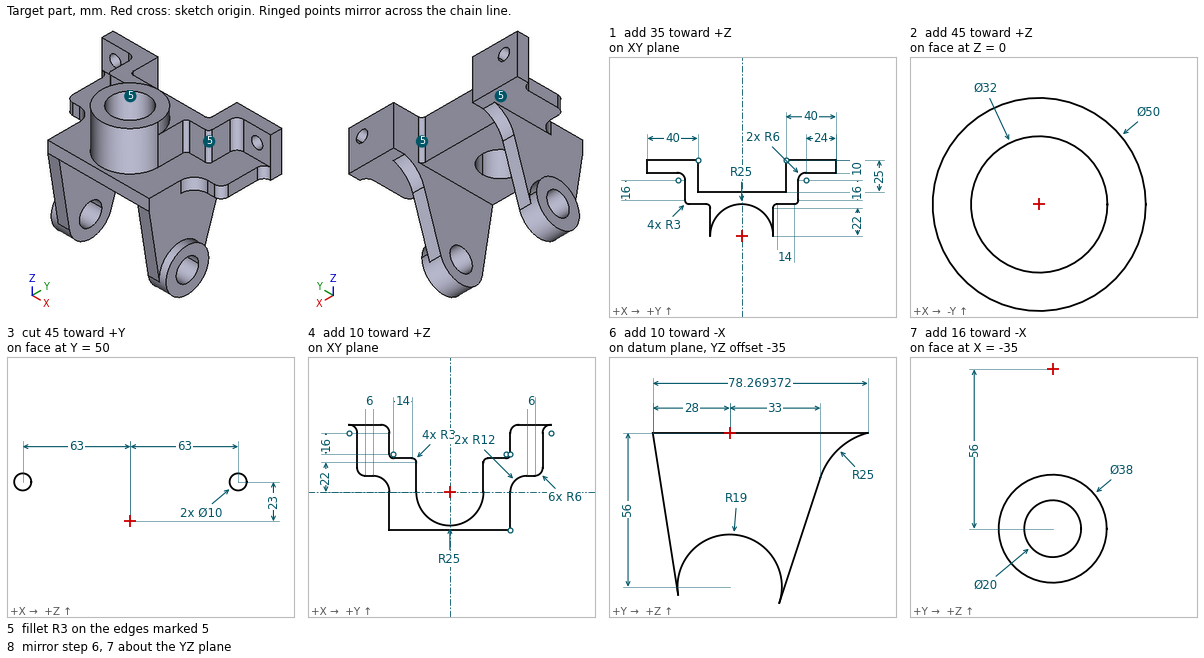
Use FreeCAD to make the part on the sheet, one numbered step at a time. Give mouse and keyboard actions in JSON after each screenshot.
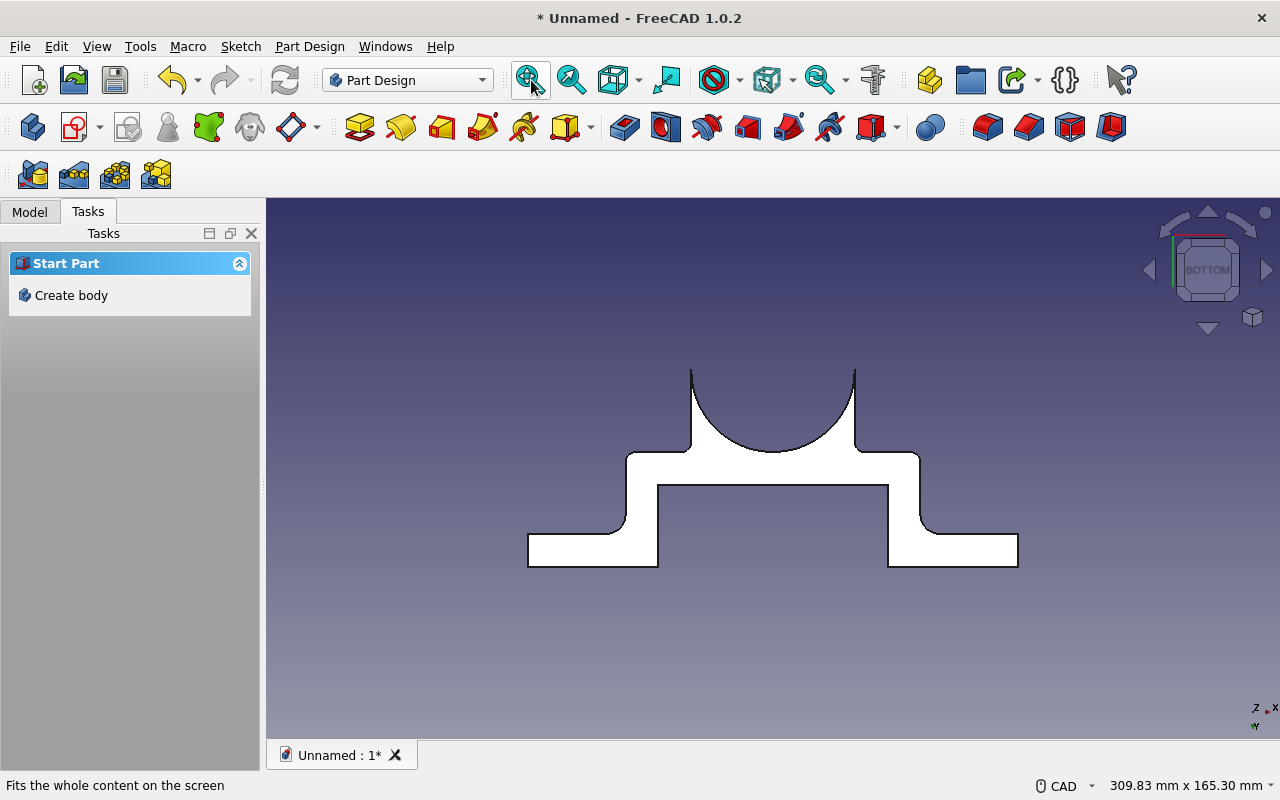
{"action": "left_click", "coordinate": [843, 467]}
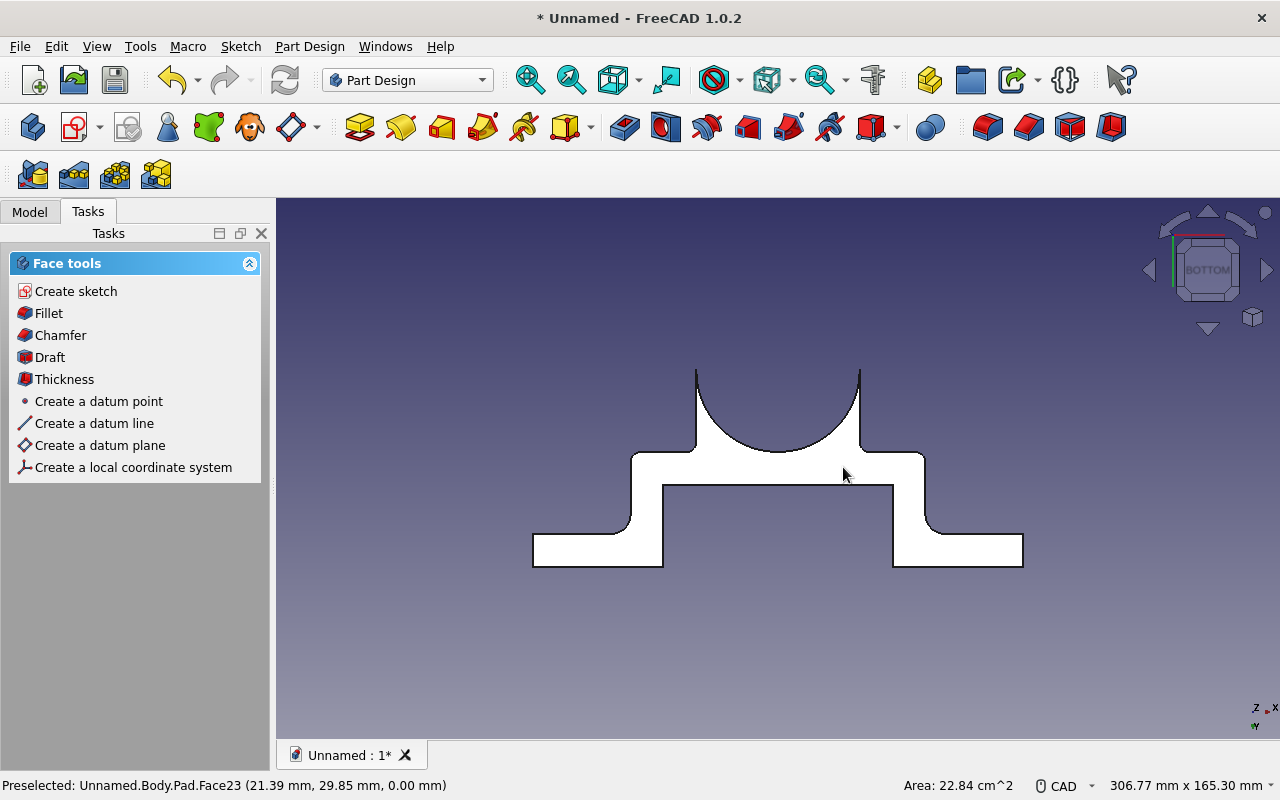
{"action": "left_click", "coordinate": [74, 128]}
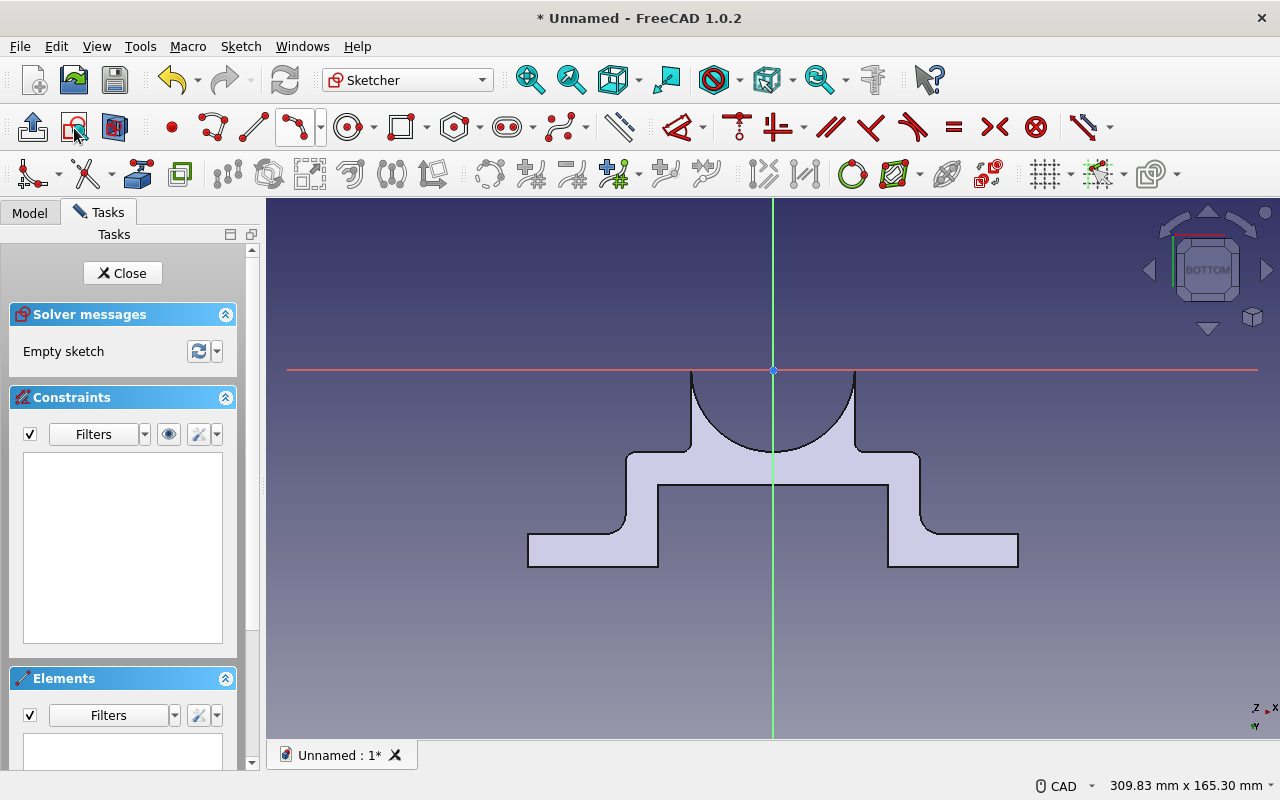
{"action": "scroll", "coordinate": [829, 290], "scroll_direction": "up", "scroll_amount": 4}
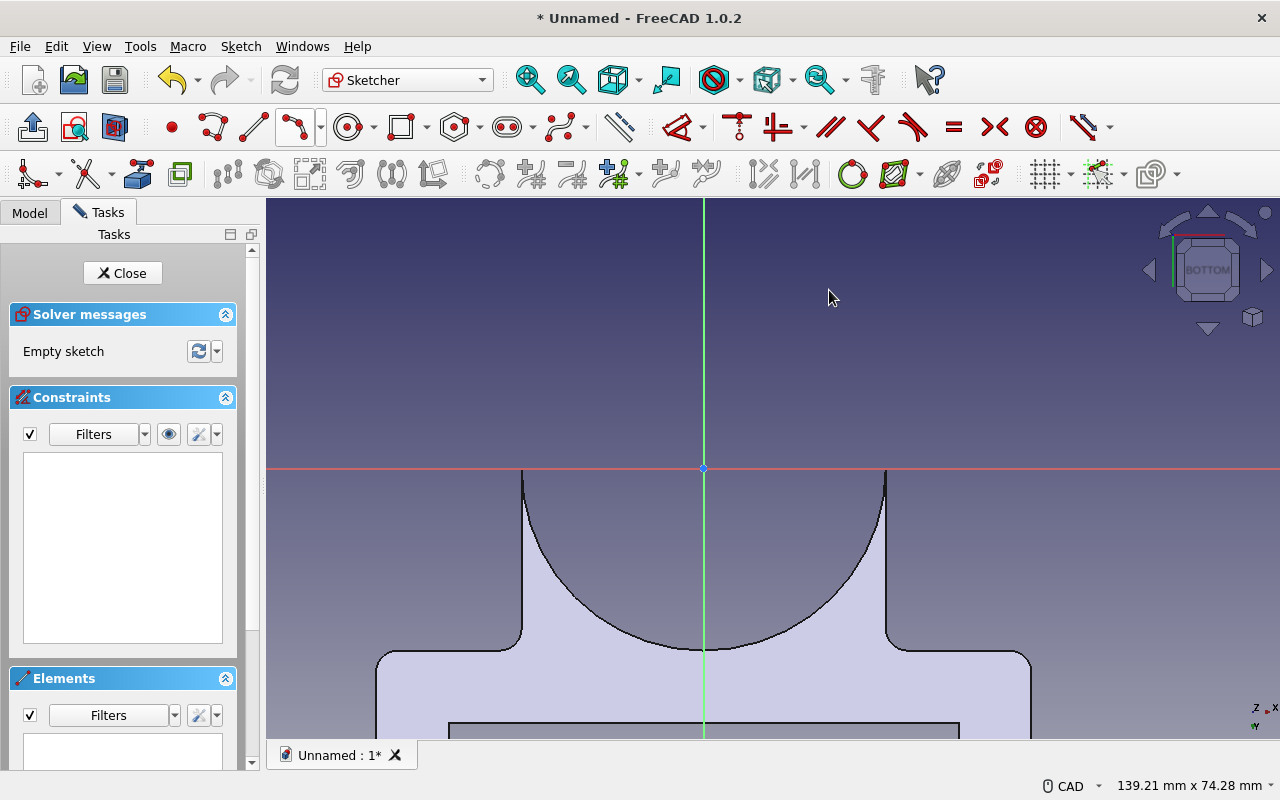
{"action": "left_click", "coordinate": [348, 128]}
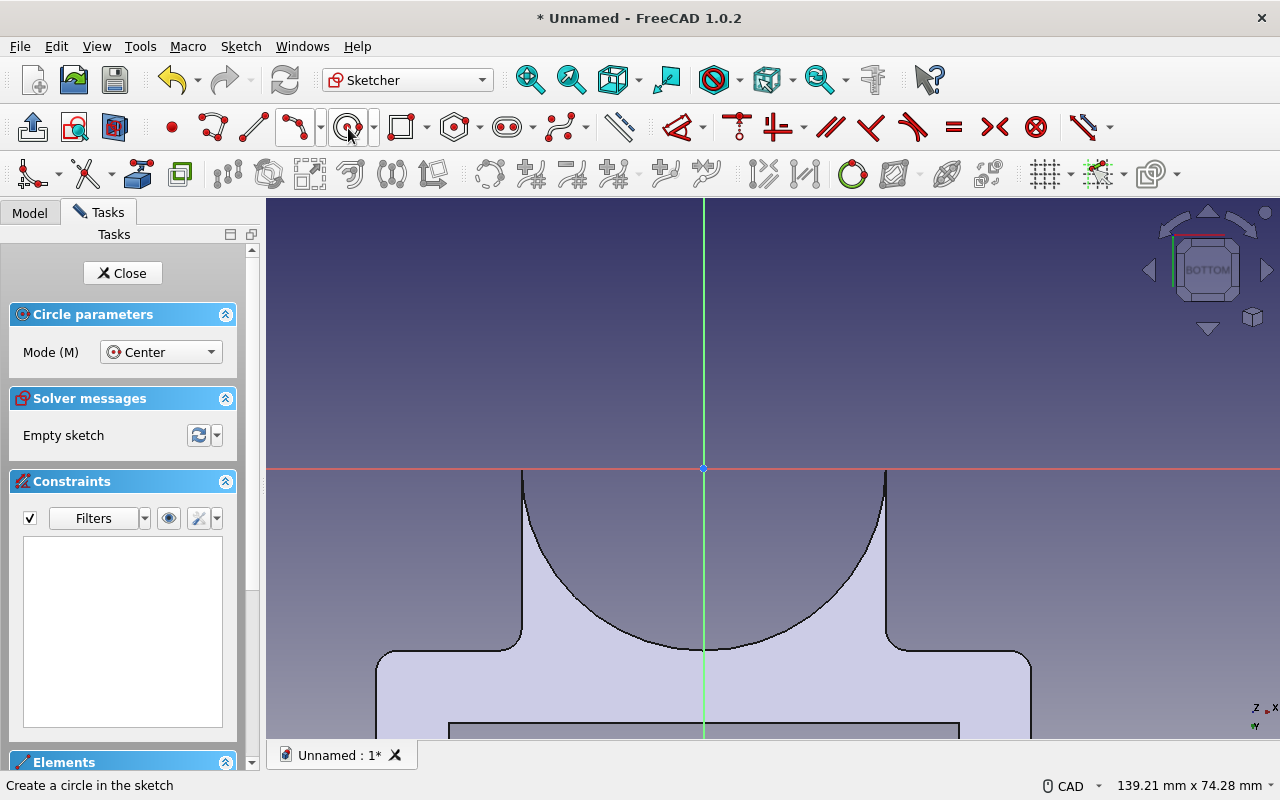
{"action": "left_click", "coordinate": [704, 469]}
{"action": "left_click", "coordinate": [832, 340]}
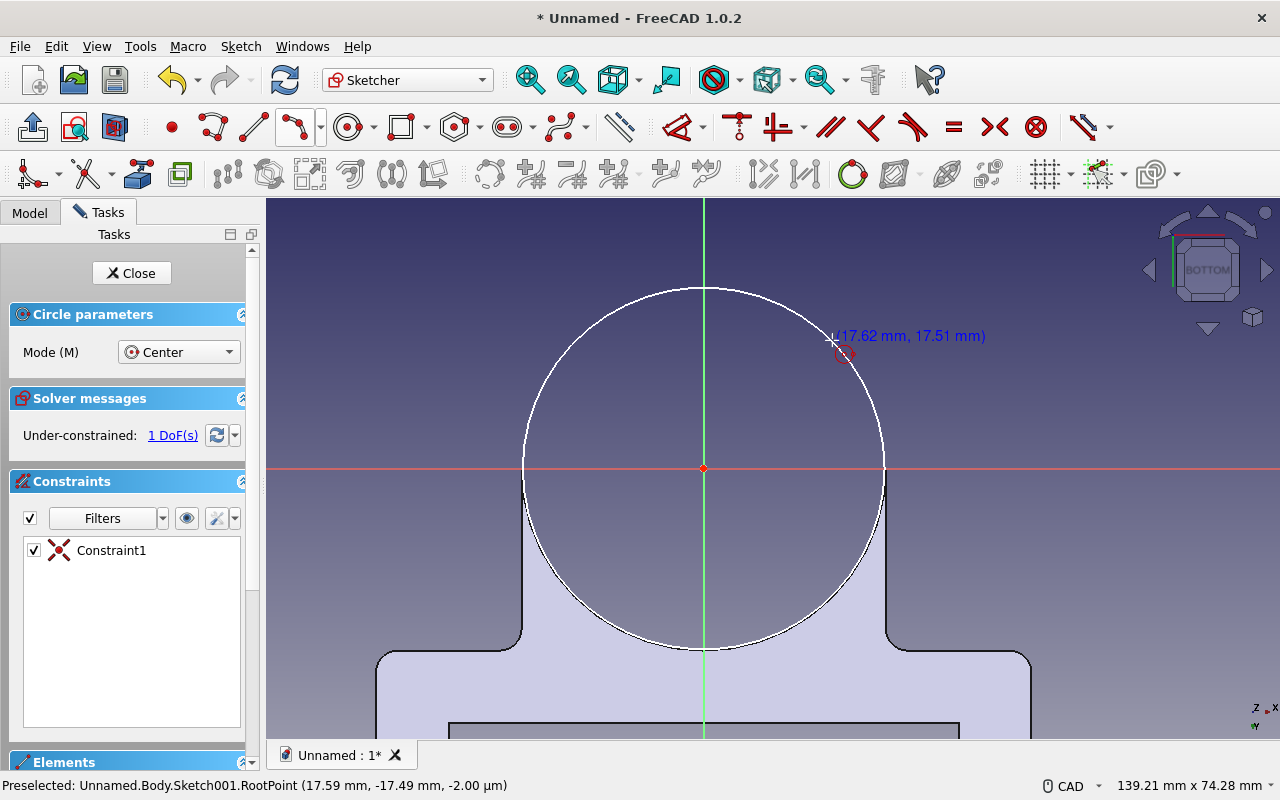
{"action": "left_click", "coordinate": [704, 469]}
{"action": "left_click", "coordinate": [786, 386]}
{"action": "key", "text": "Escape"}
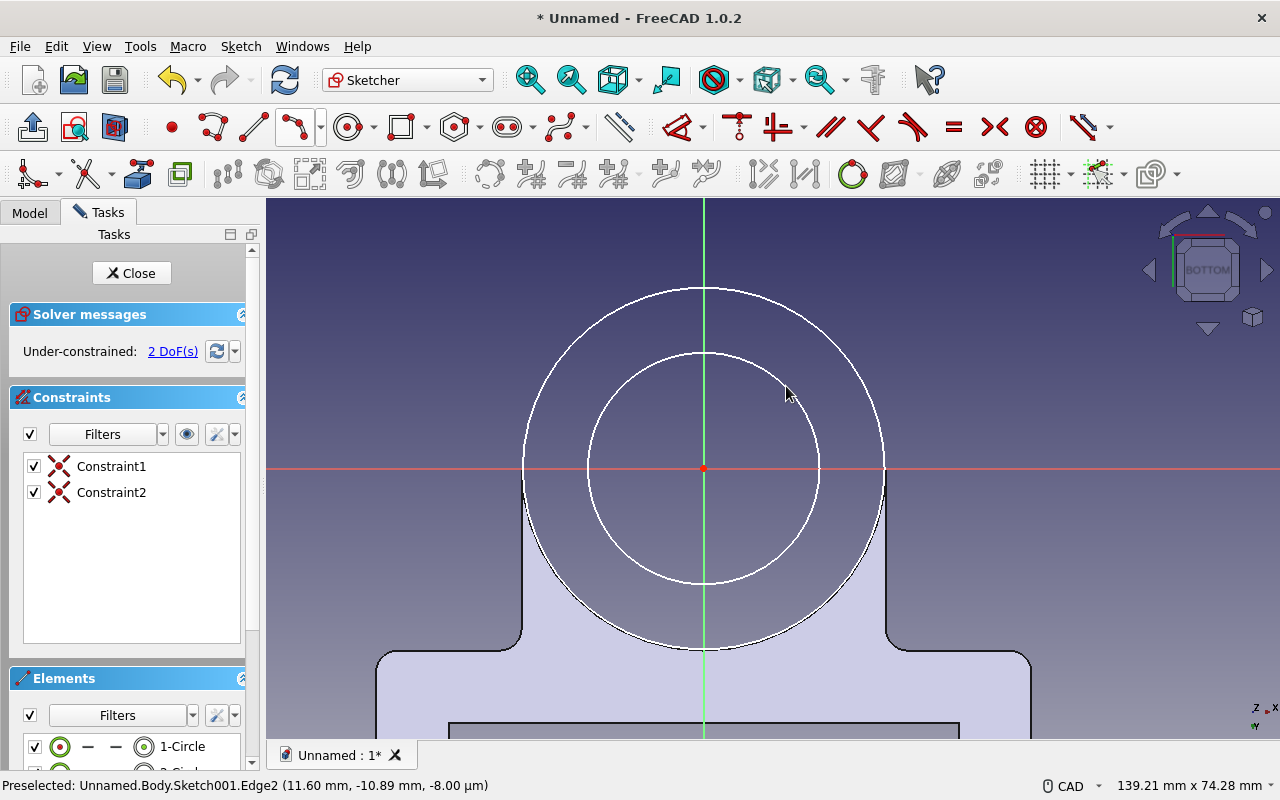
{"action": "left_click", "coordinate": [676, 128]}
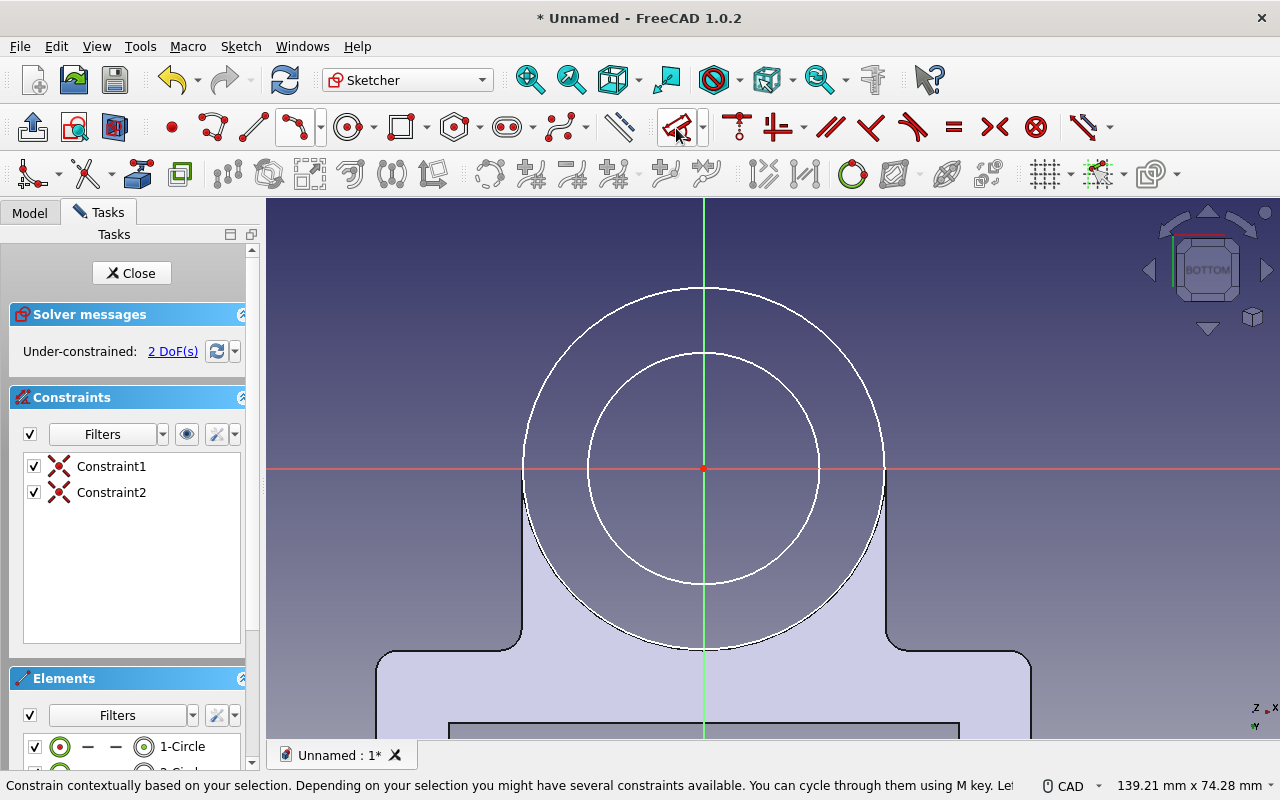
{"action": "left_click", "coordinate": [831, 340]}
{"action": "left_click", "coordinate": [854, 317]}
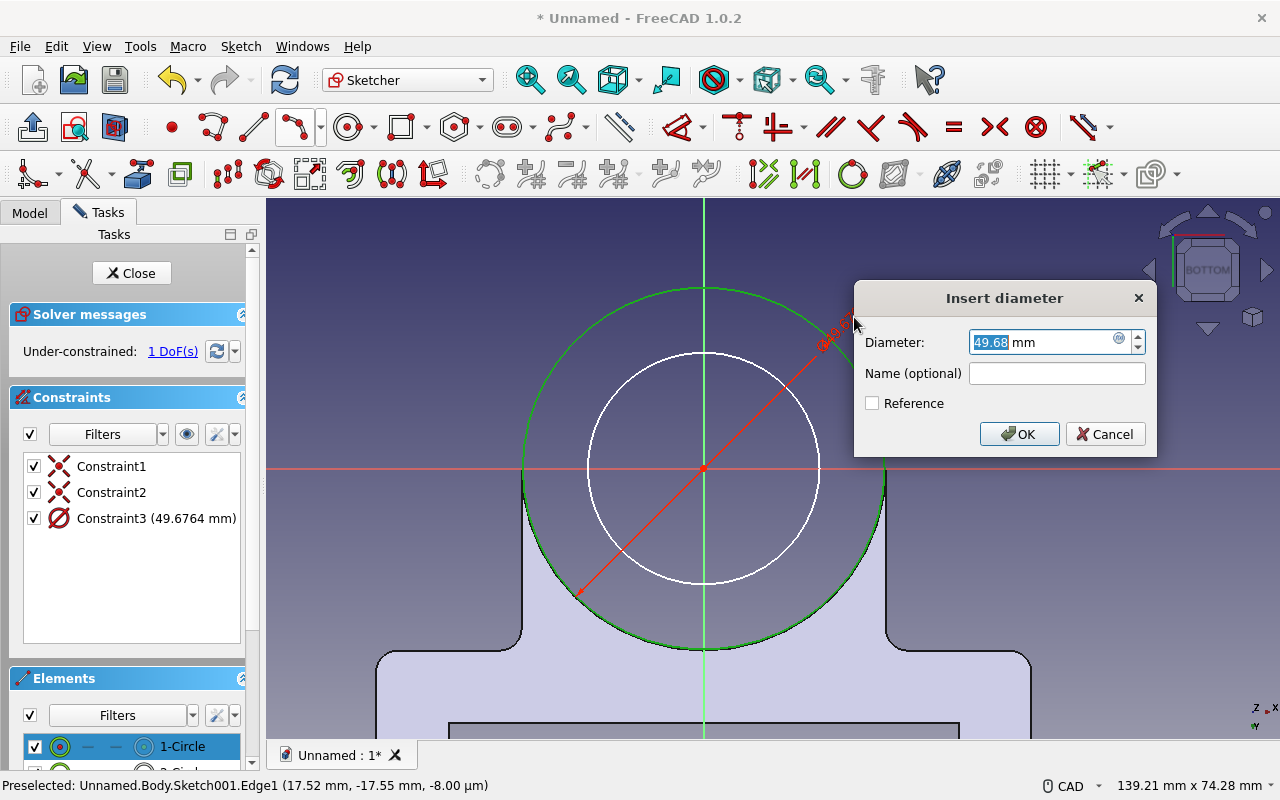
{"action": "type", "text": "50"}
{"action": "key", "text": "Return"}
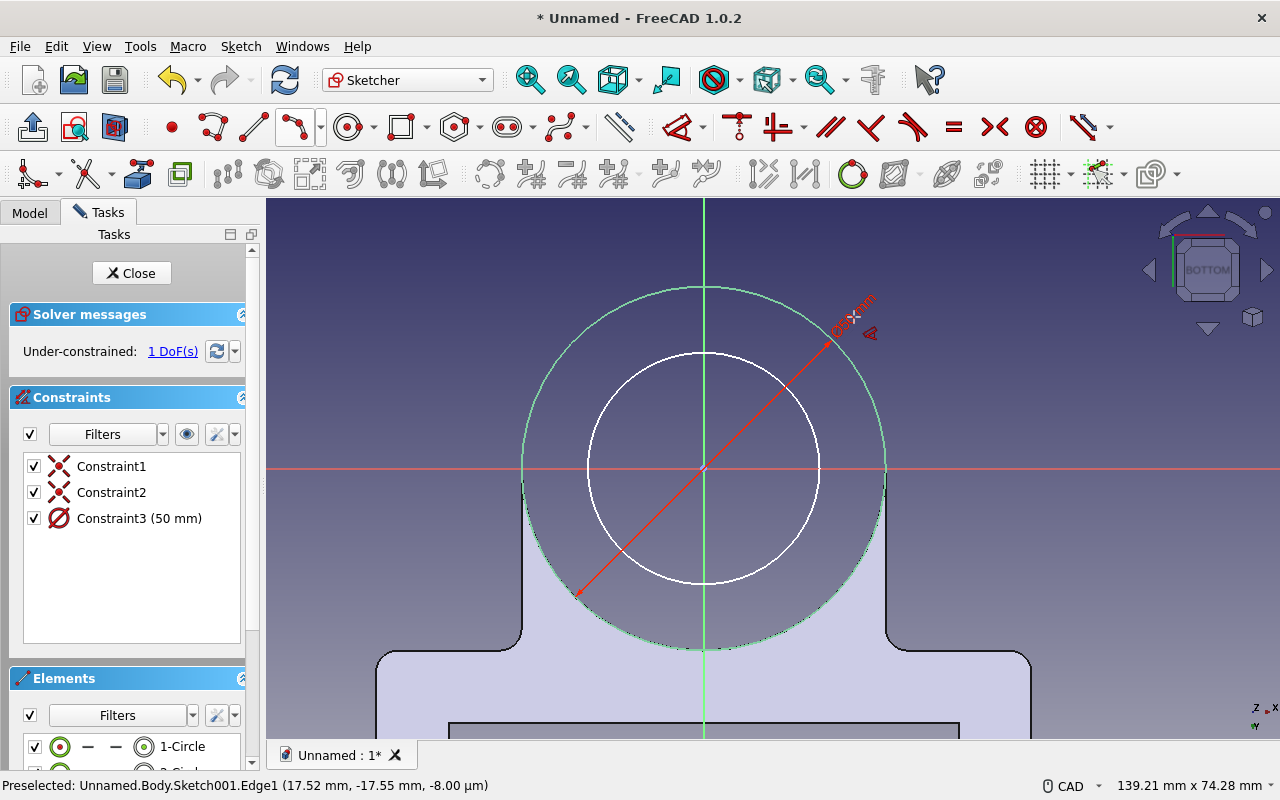
{"action": "left_click", "coordinate": [785, 386]}
{"action": "left_click", "coordinate": [807, 363]}